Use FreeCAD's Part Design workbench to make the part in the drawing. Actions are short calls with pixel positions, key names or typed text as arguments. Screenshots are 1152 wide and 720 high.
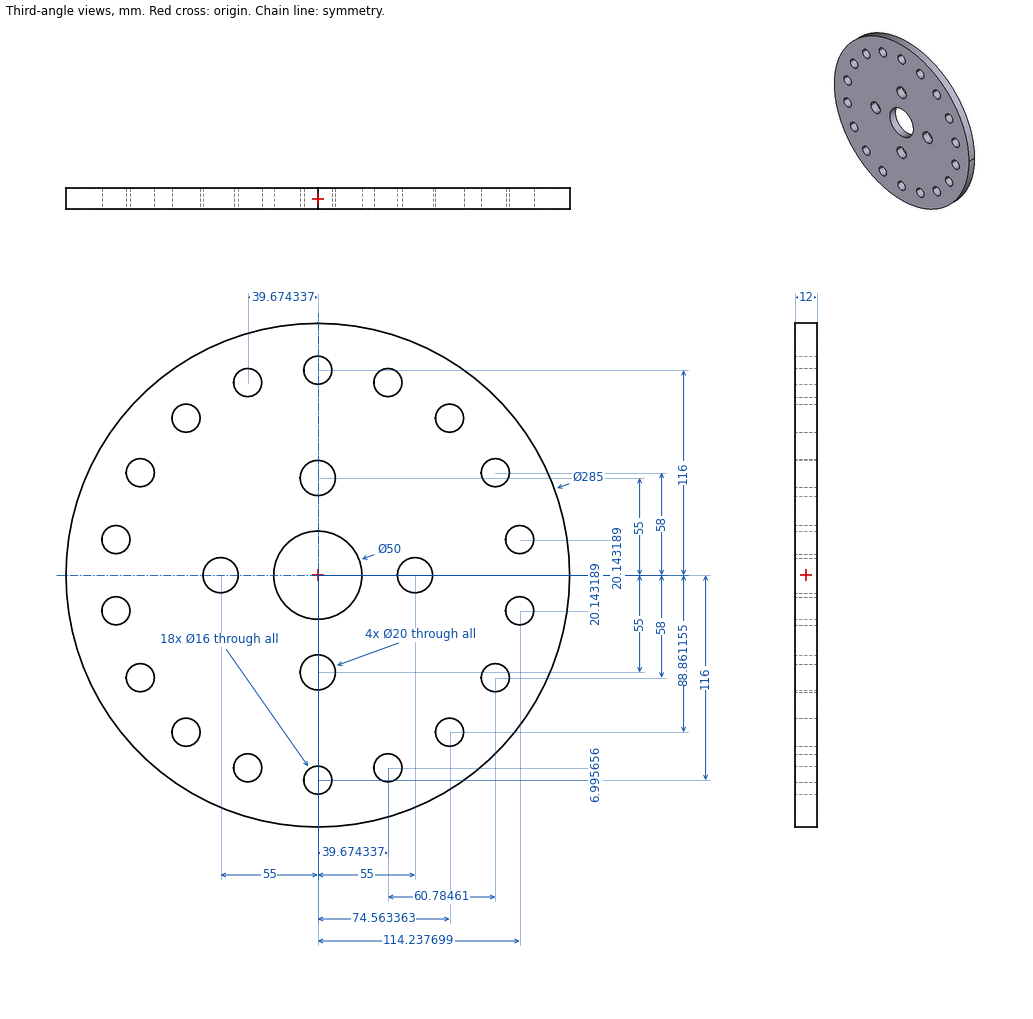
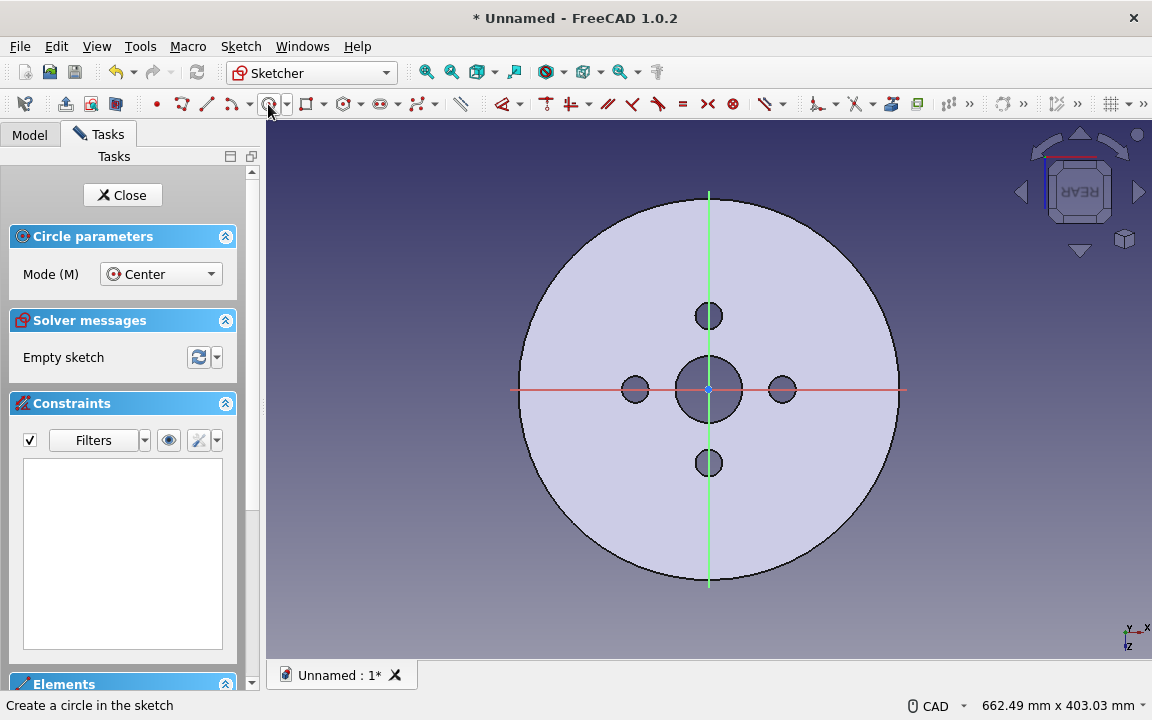
scroll(709, 234, up, 4)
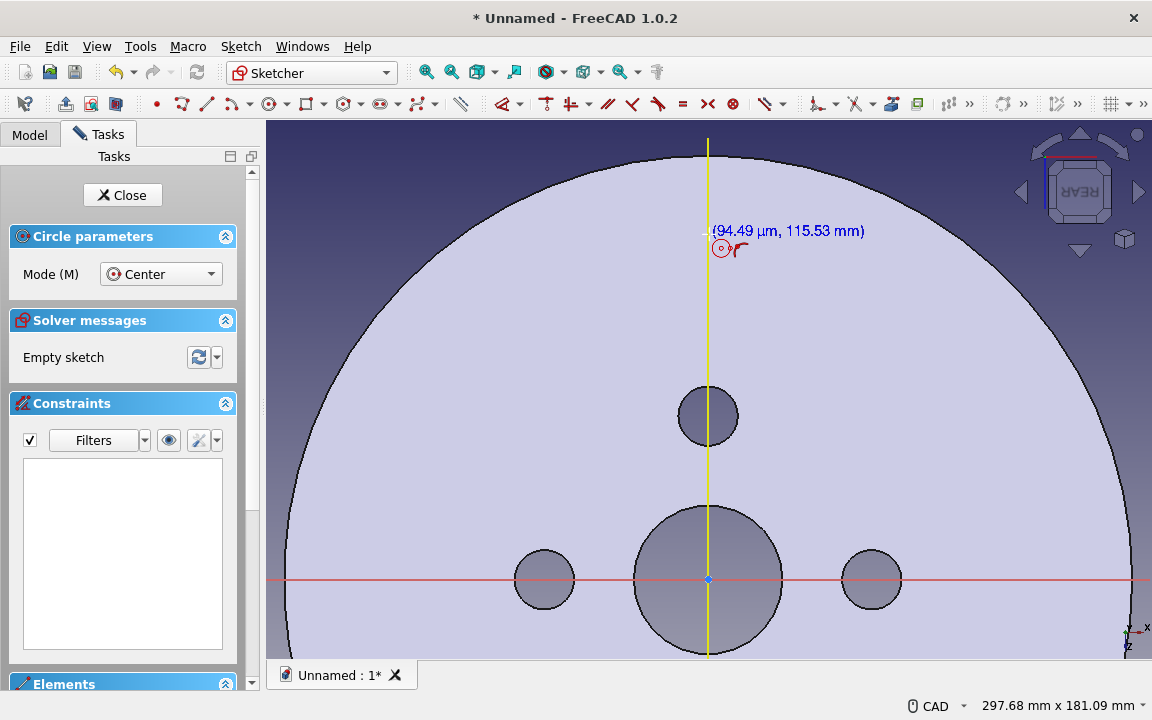
click(708, 235)
move(725, 218)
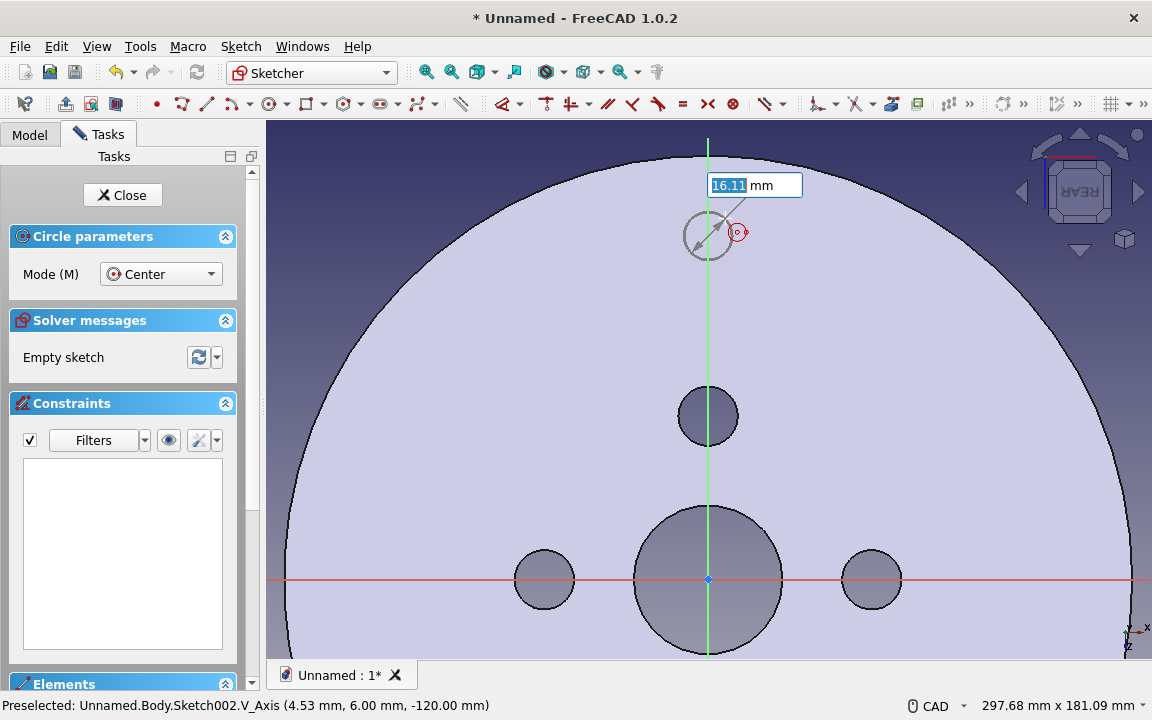
text(16)
key(Return)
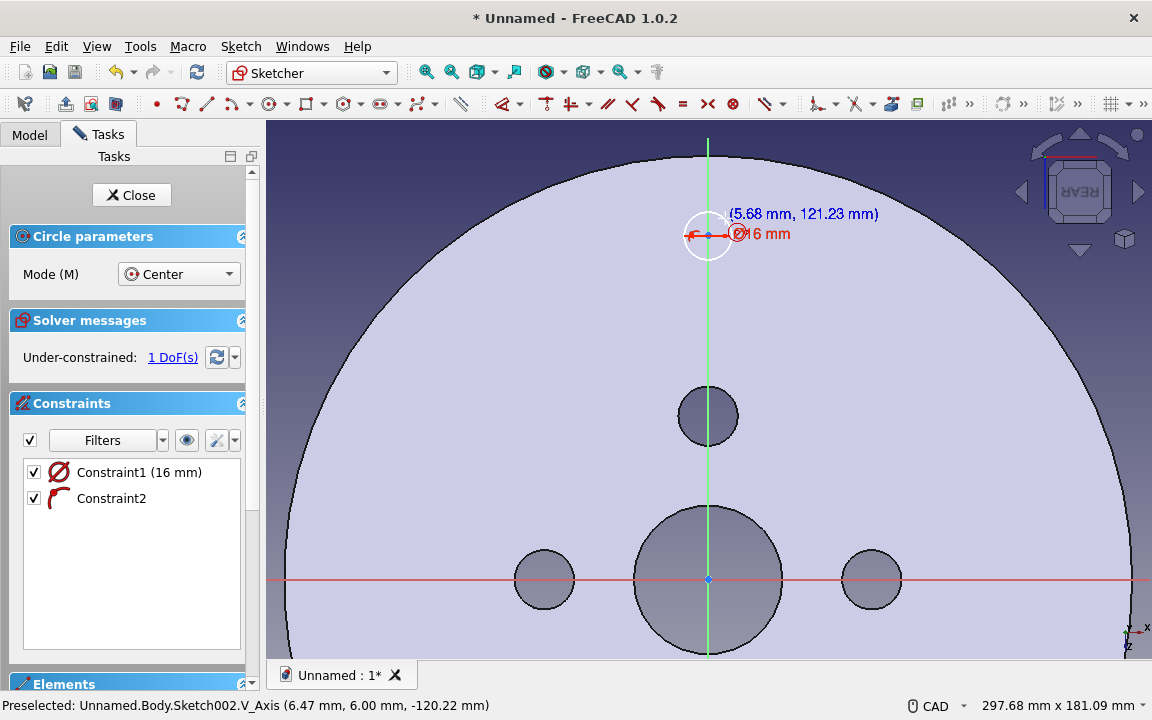
click(826, 255)
move(843, 239)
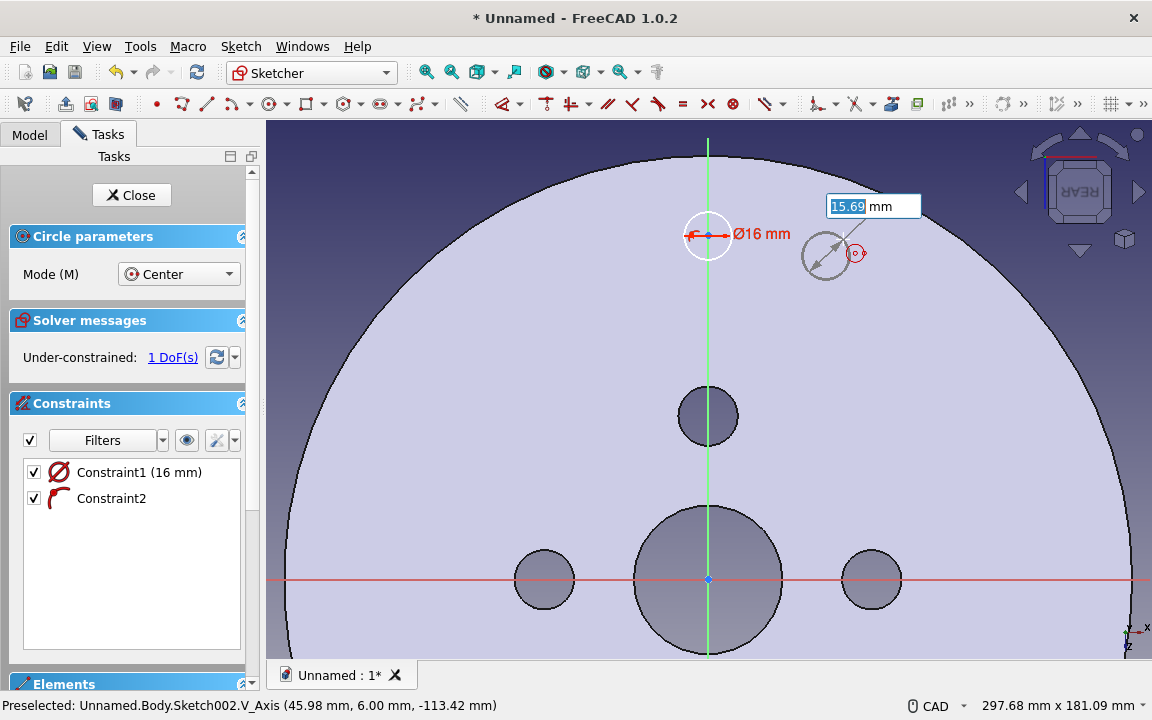
text(16)
key(Return)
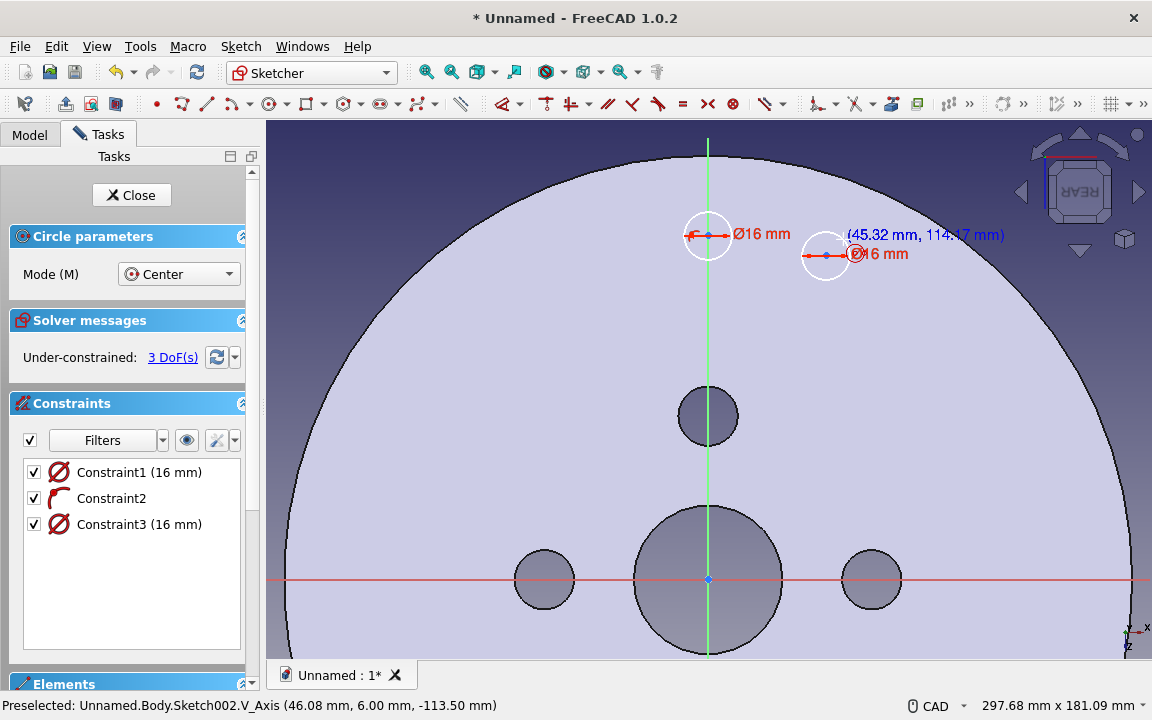
click(930, 315)
move(947, 298)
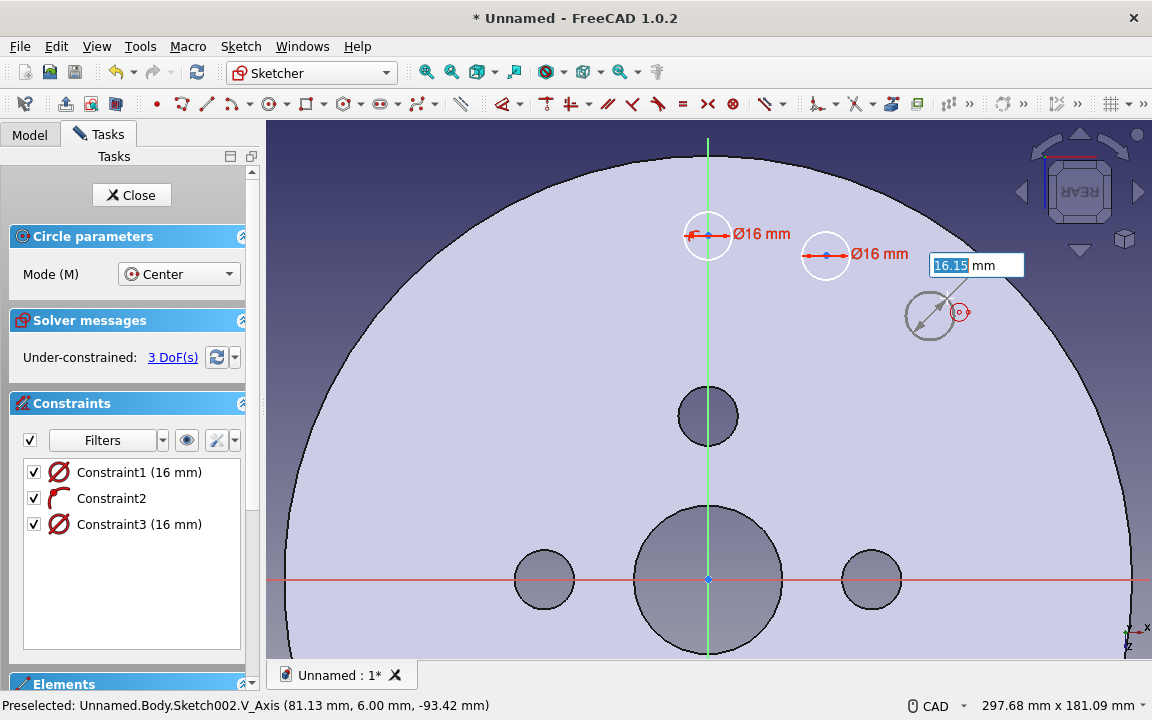
text(16)
key(Return)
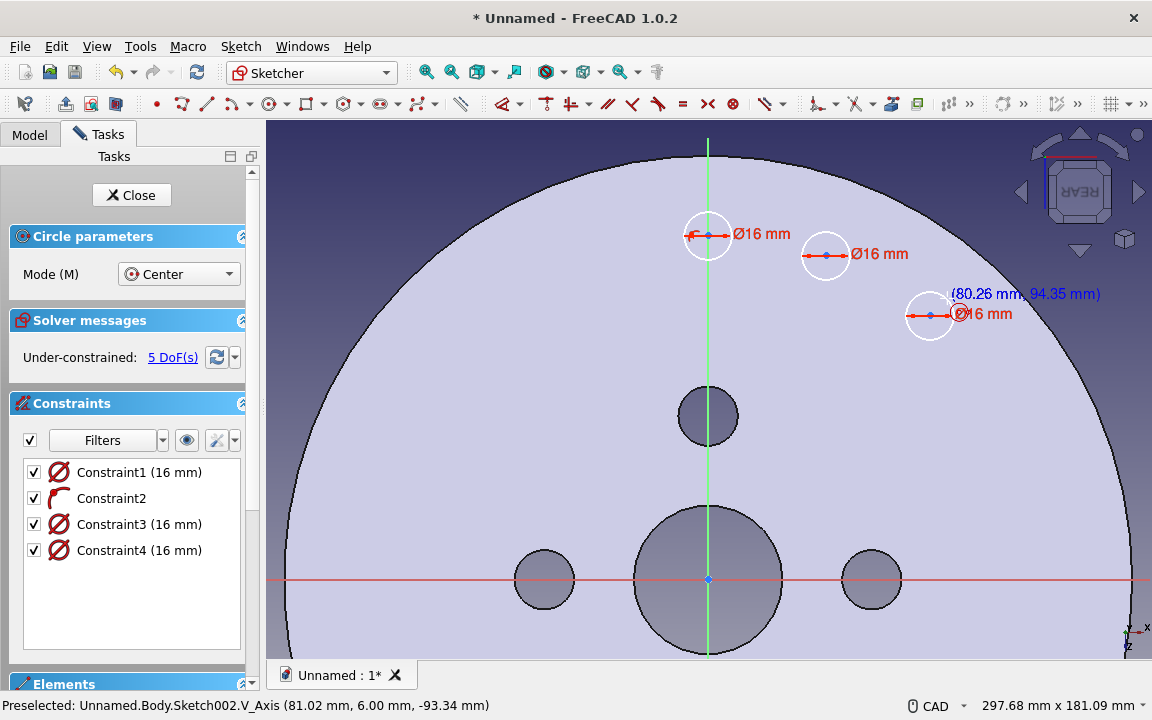
scroll(585, 234, down, 4)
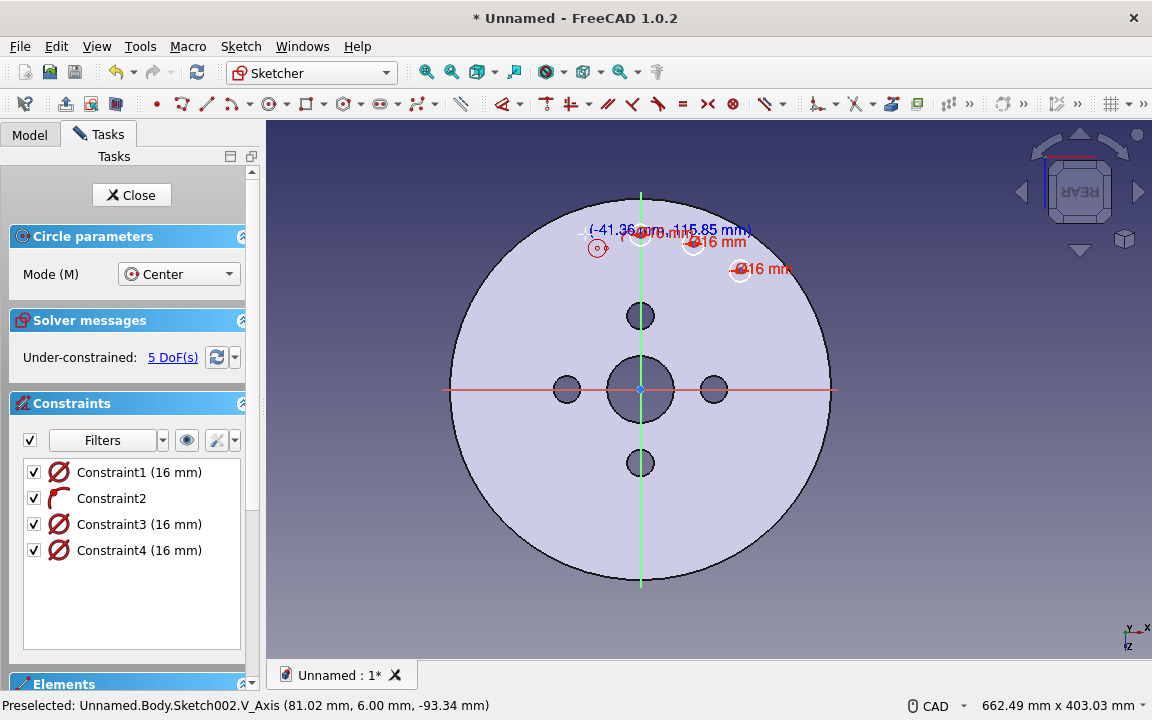
scroll(775, 312, up, 4)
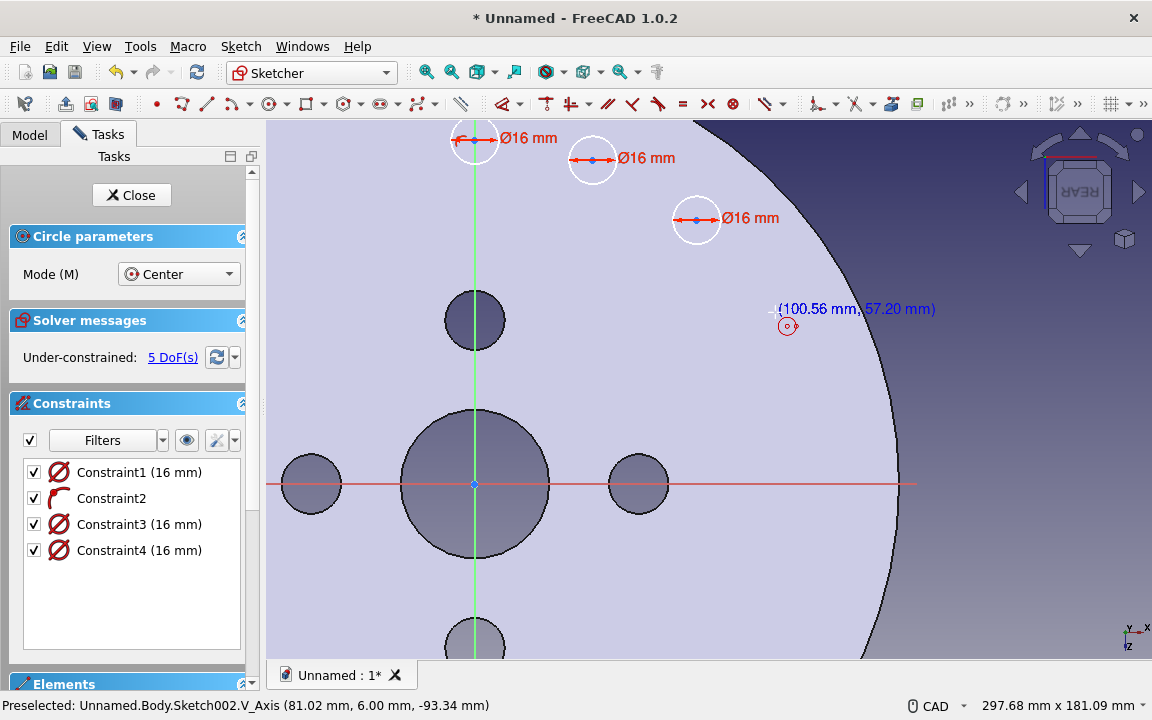
click(774, 311)
move(791, 295)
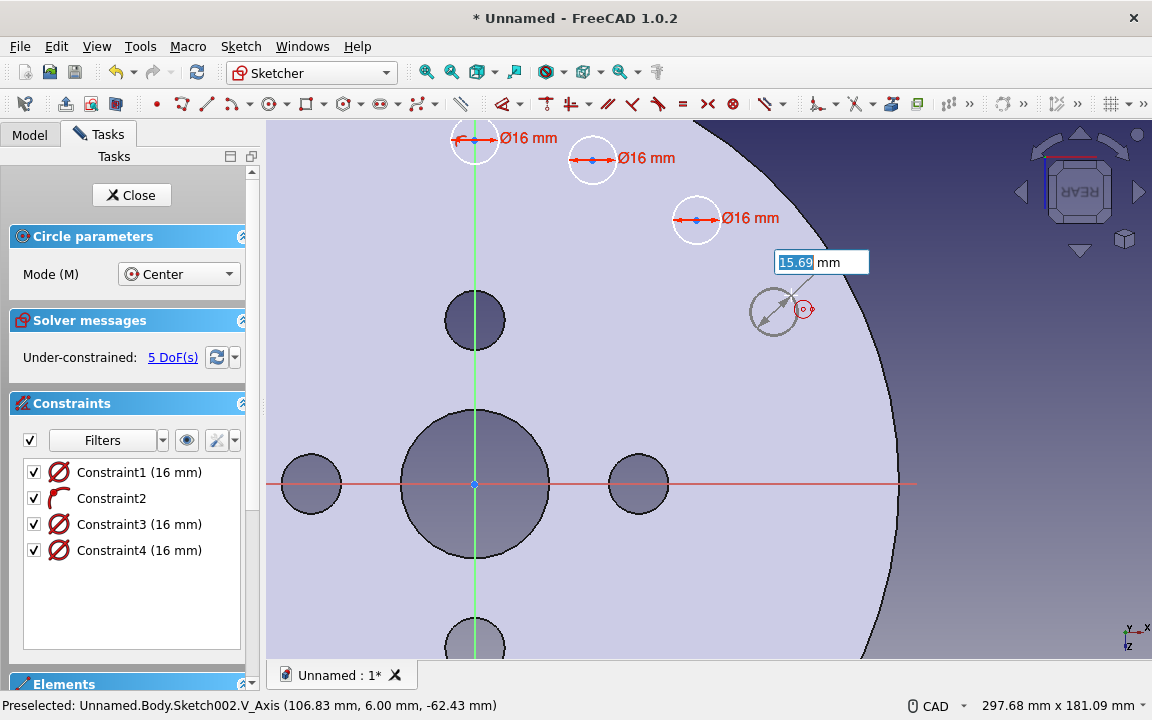
text(16)
key(Return)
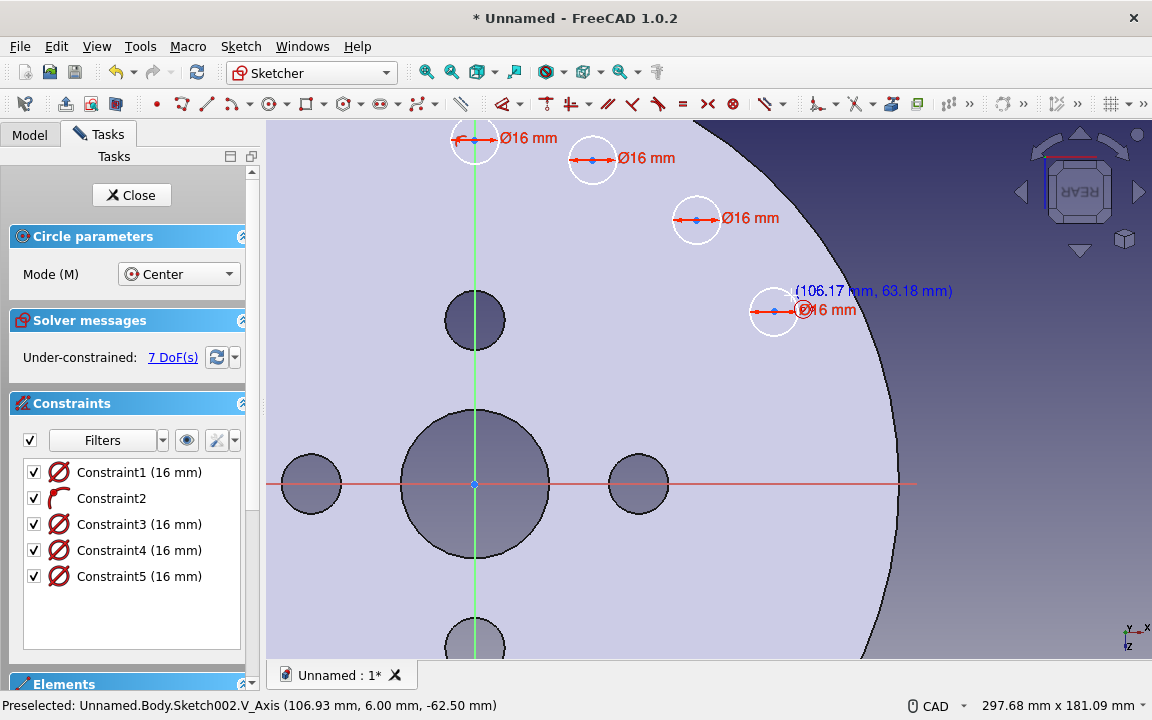
click(815, 424)
move(832, 407)